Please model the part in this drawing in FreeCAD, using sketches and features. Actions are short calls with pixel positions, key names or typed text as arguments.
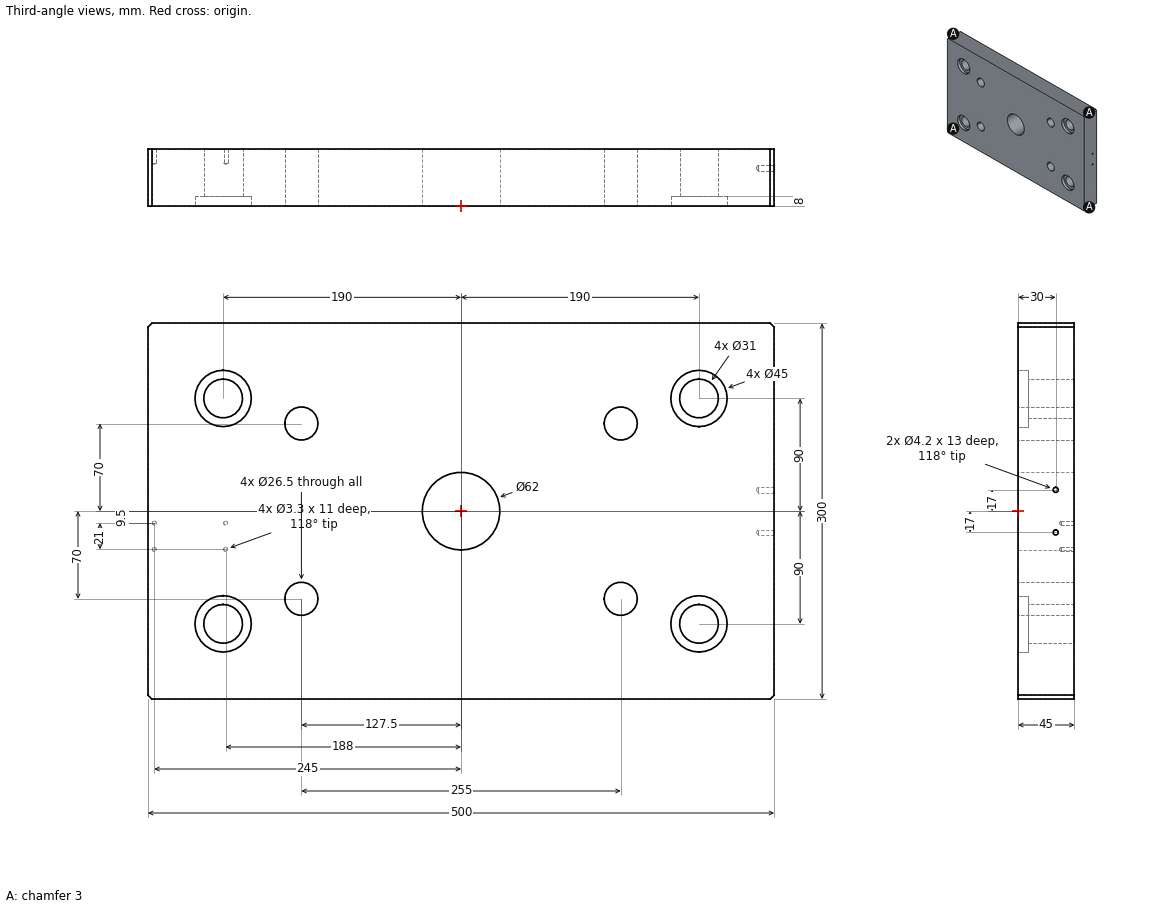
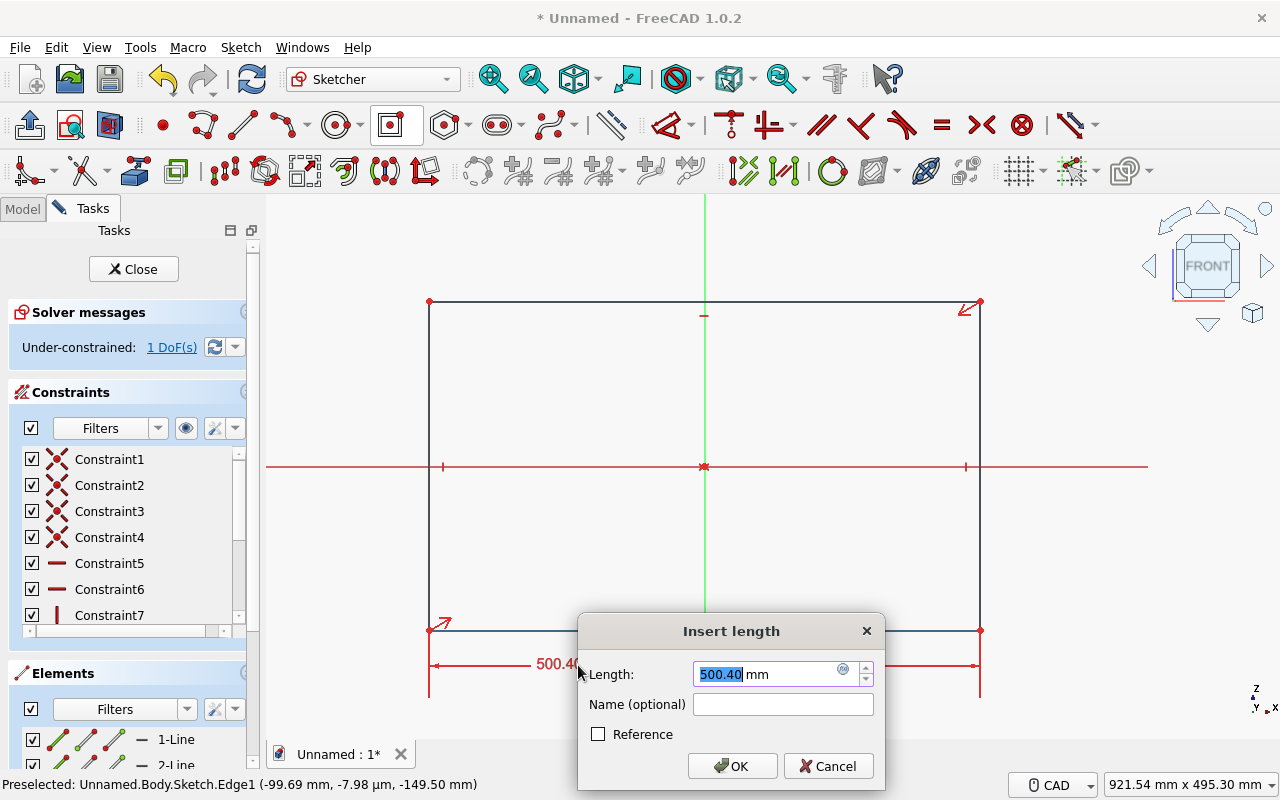
text(500)
key(Return)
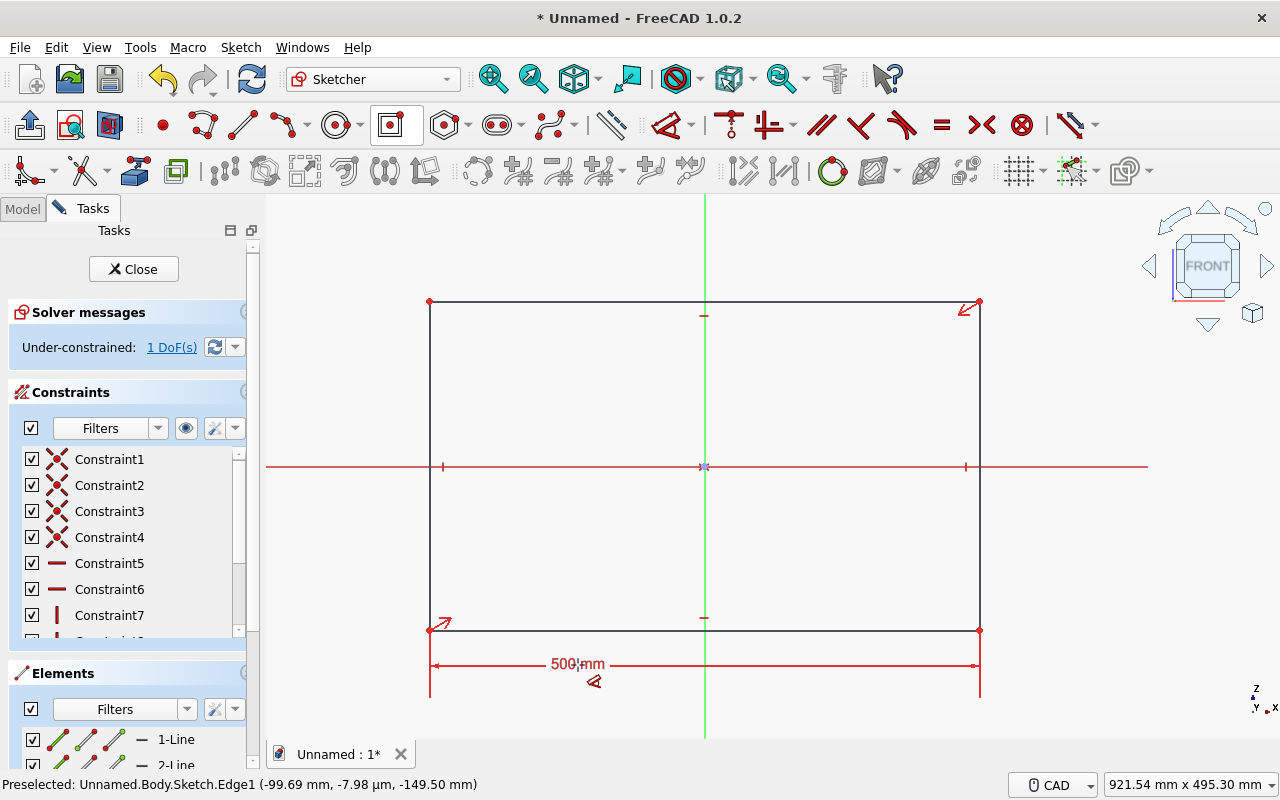
click(980, 532)
click(1014, 391)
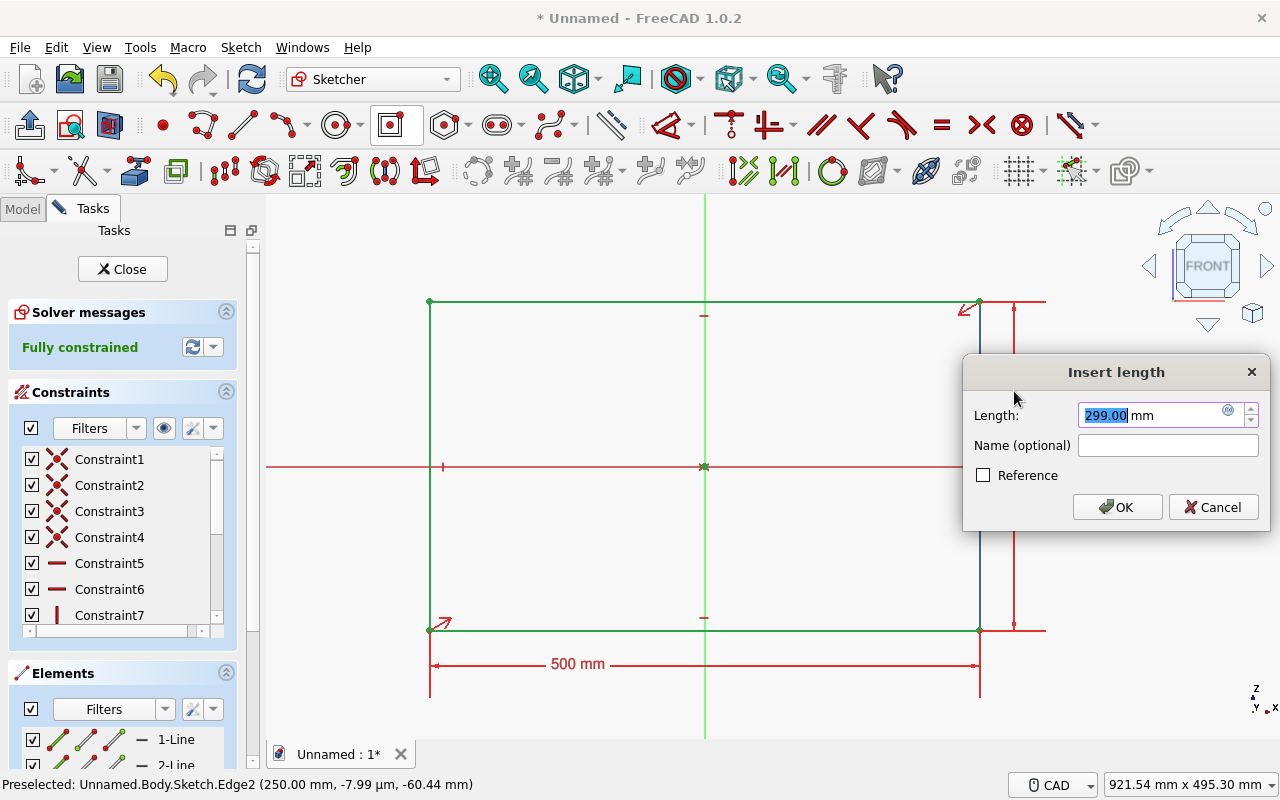
text(300)
key(Return)
key(Escape)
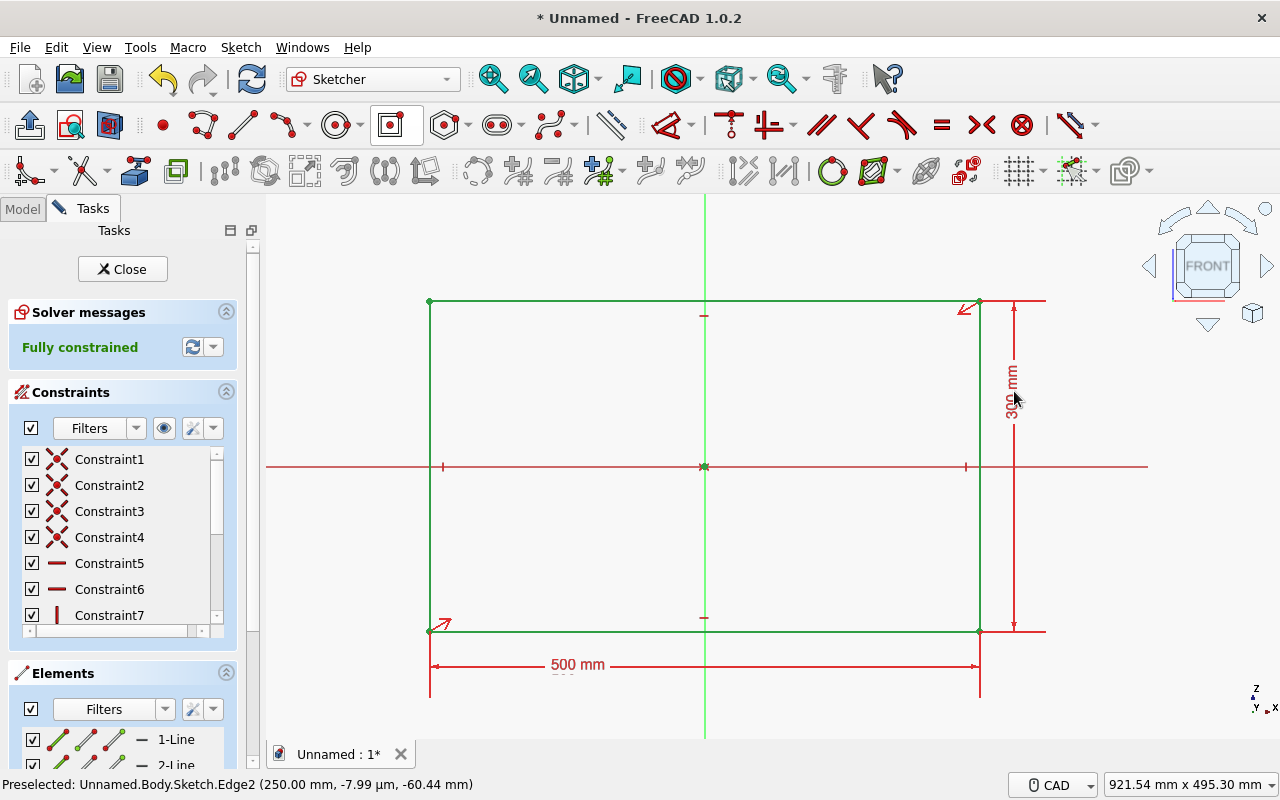
click(123, 269)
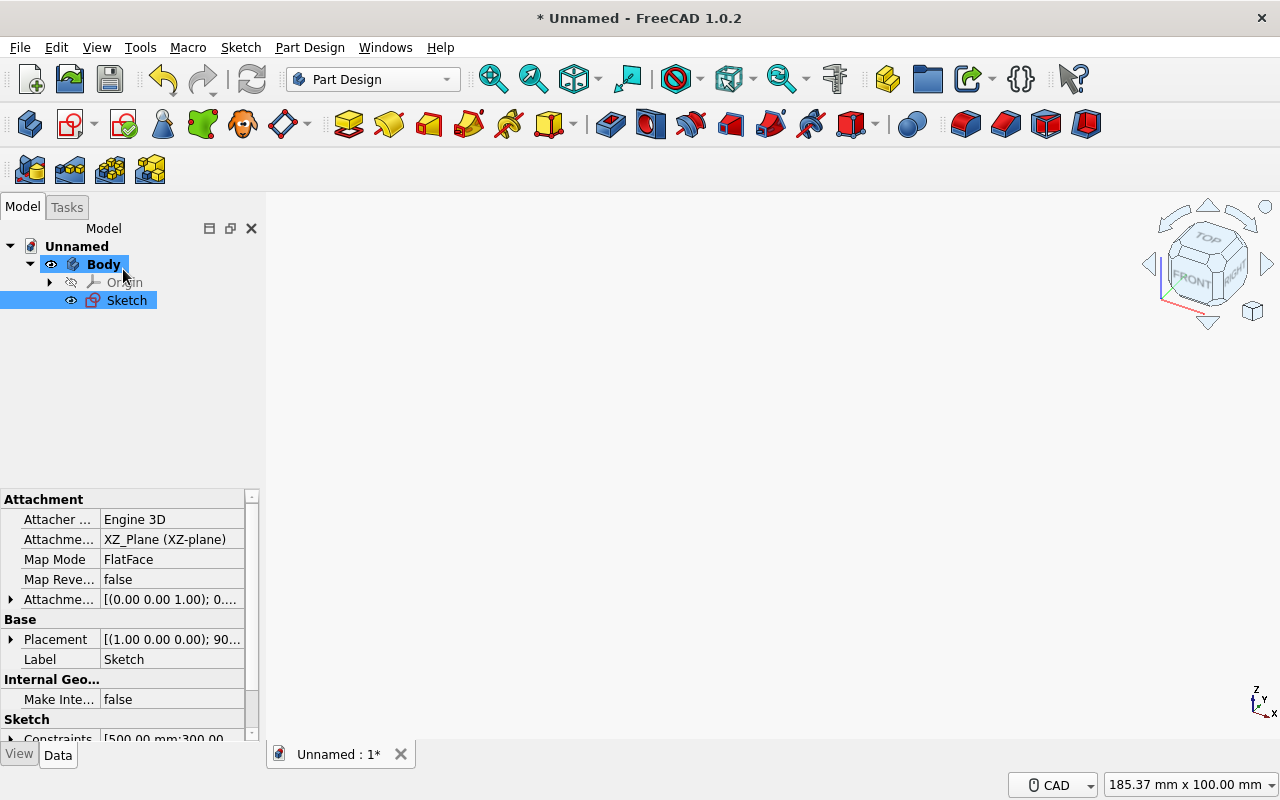
click(350, 124)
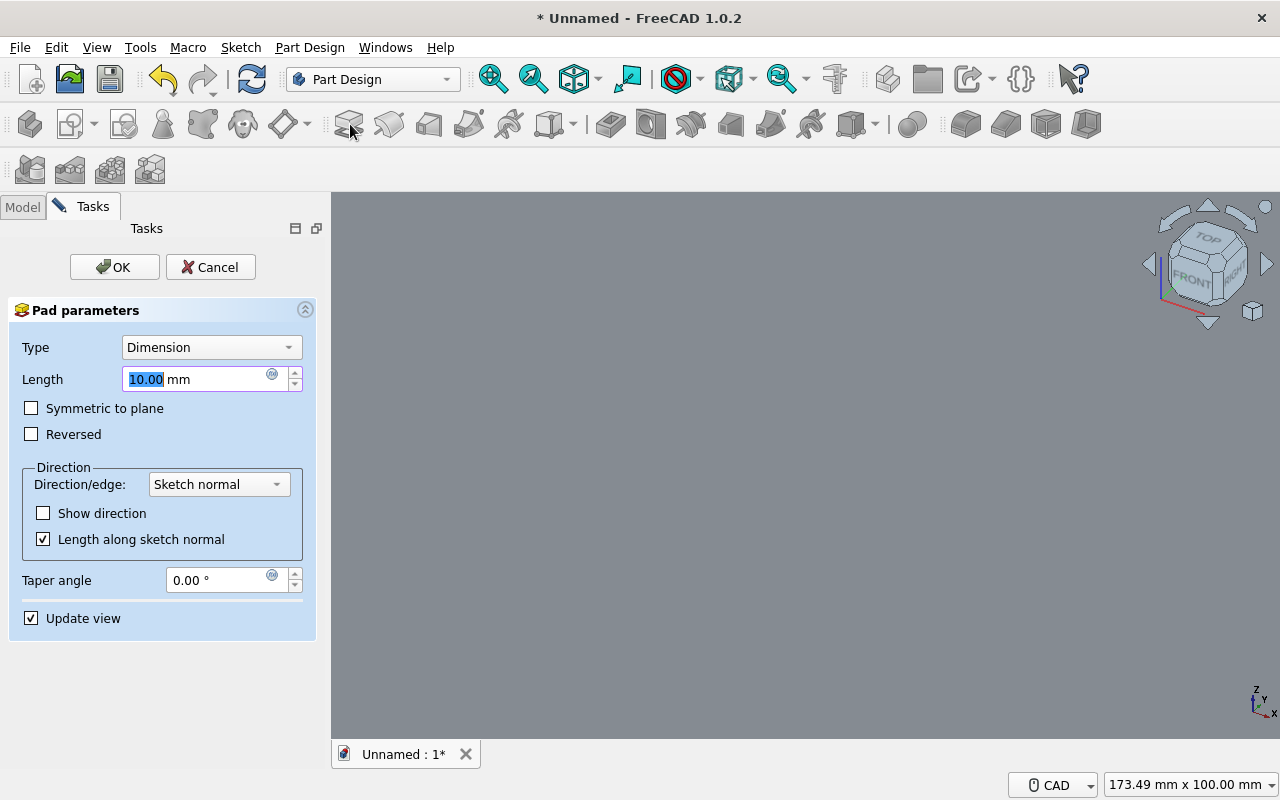
text(45)
key(Tab)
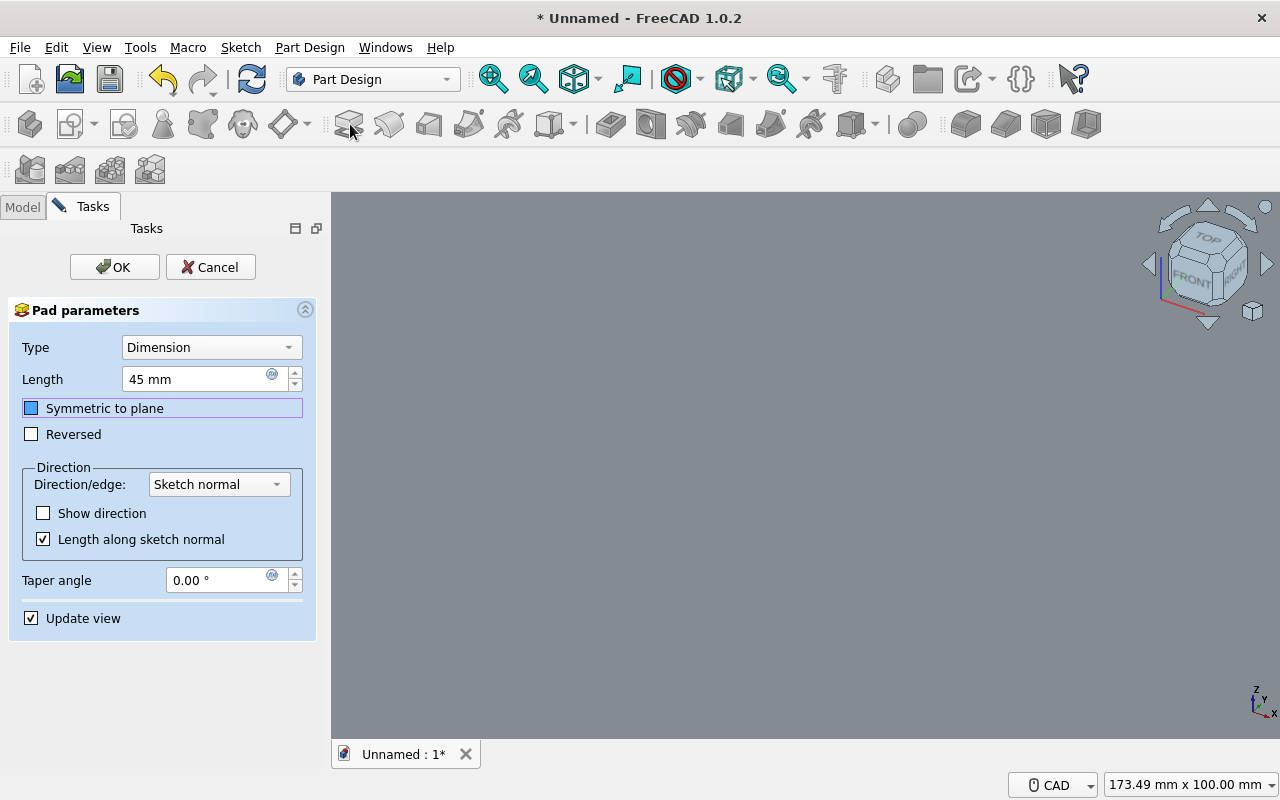
click(30, 434)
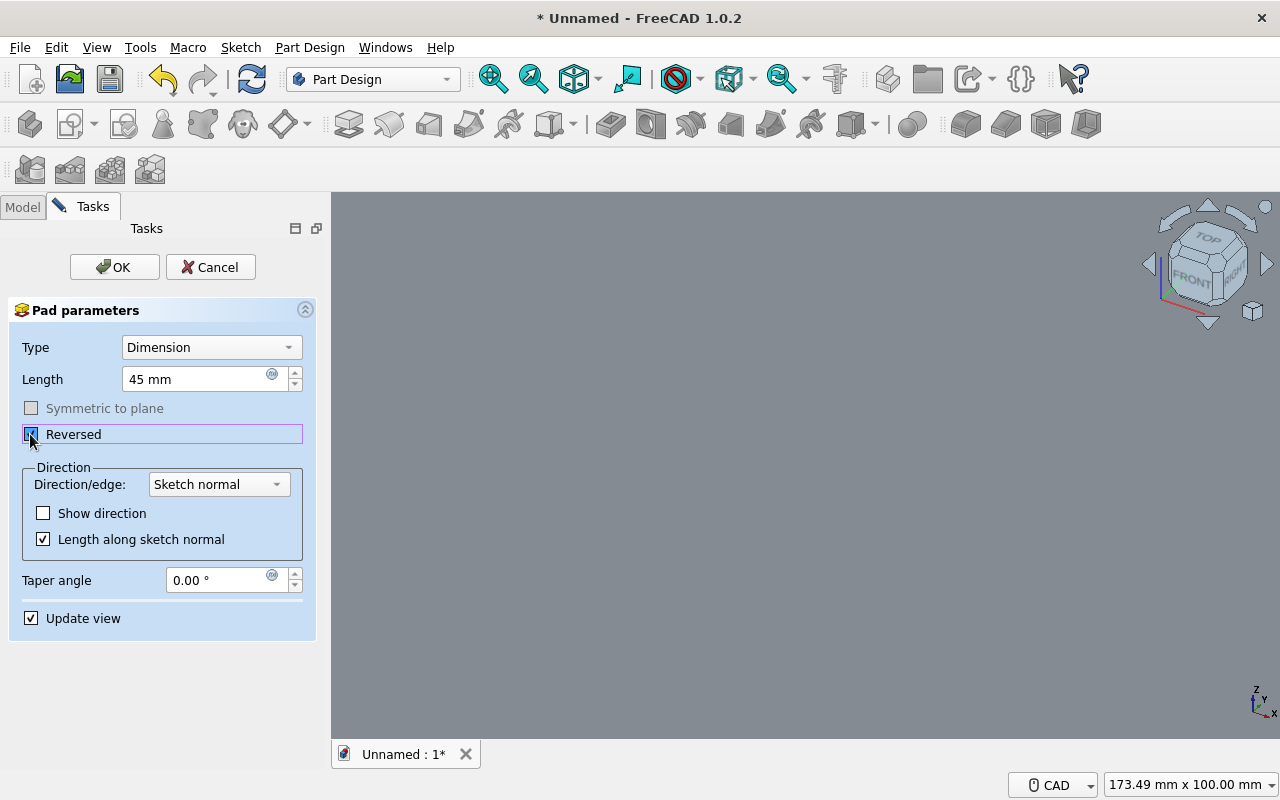
click(115, 267)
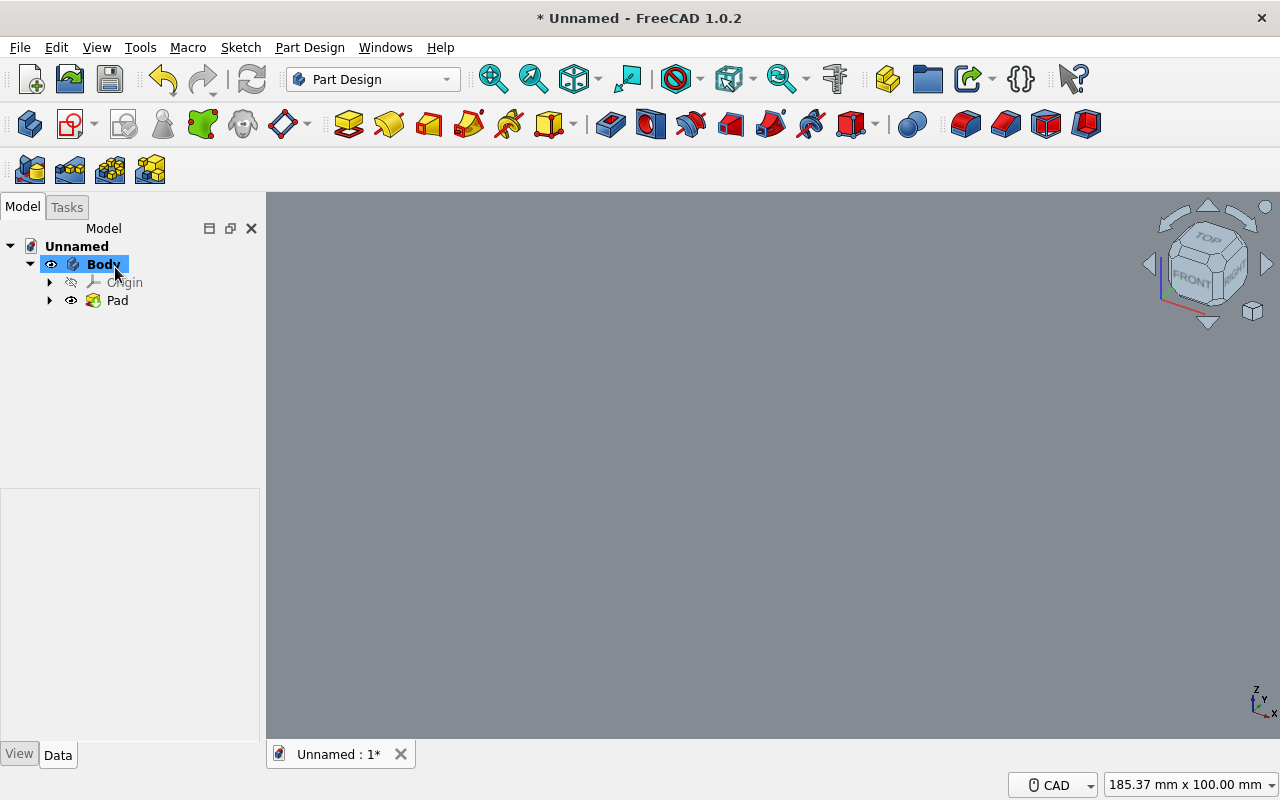
click(494, 80)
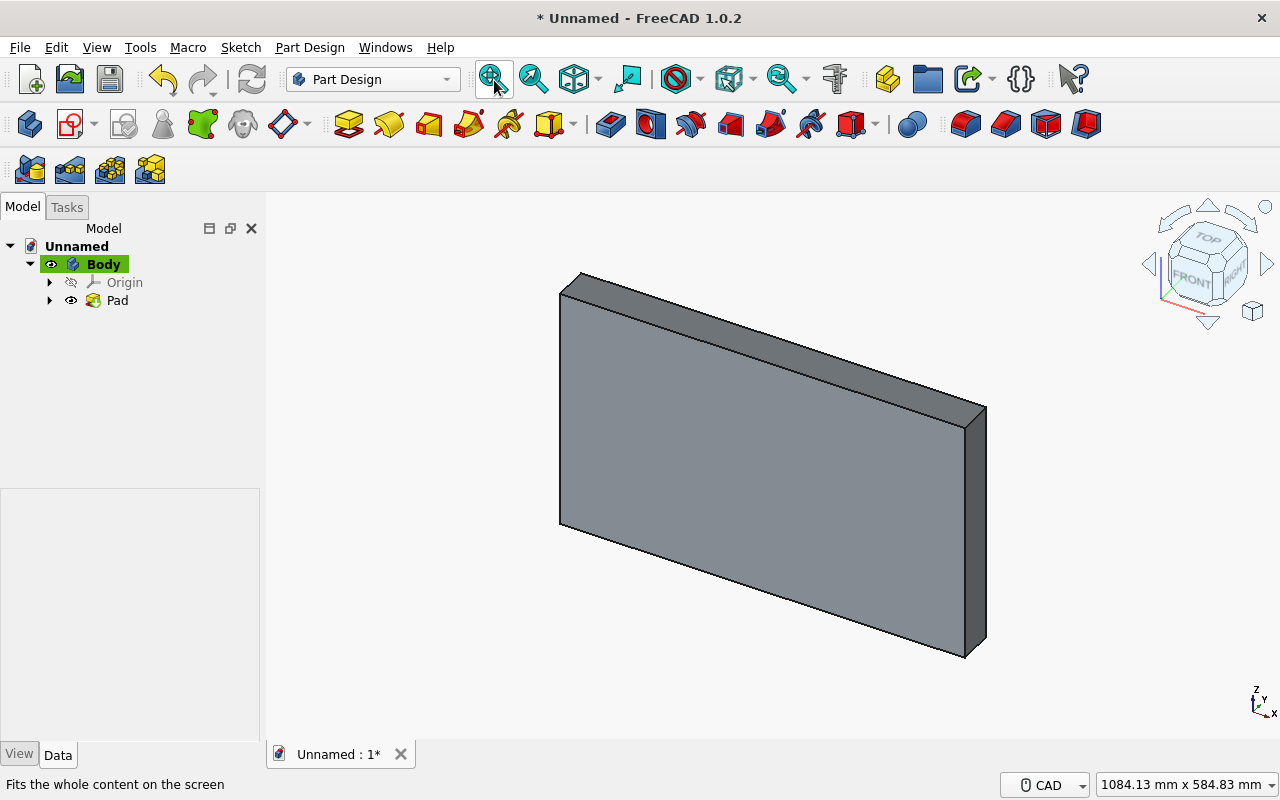
click(820, 494)